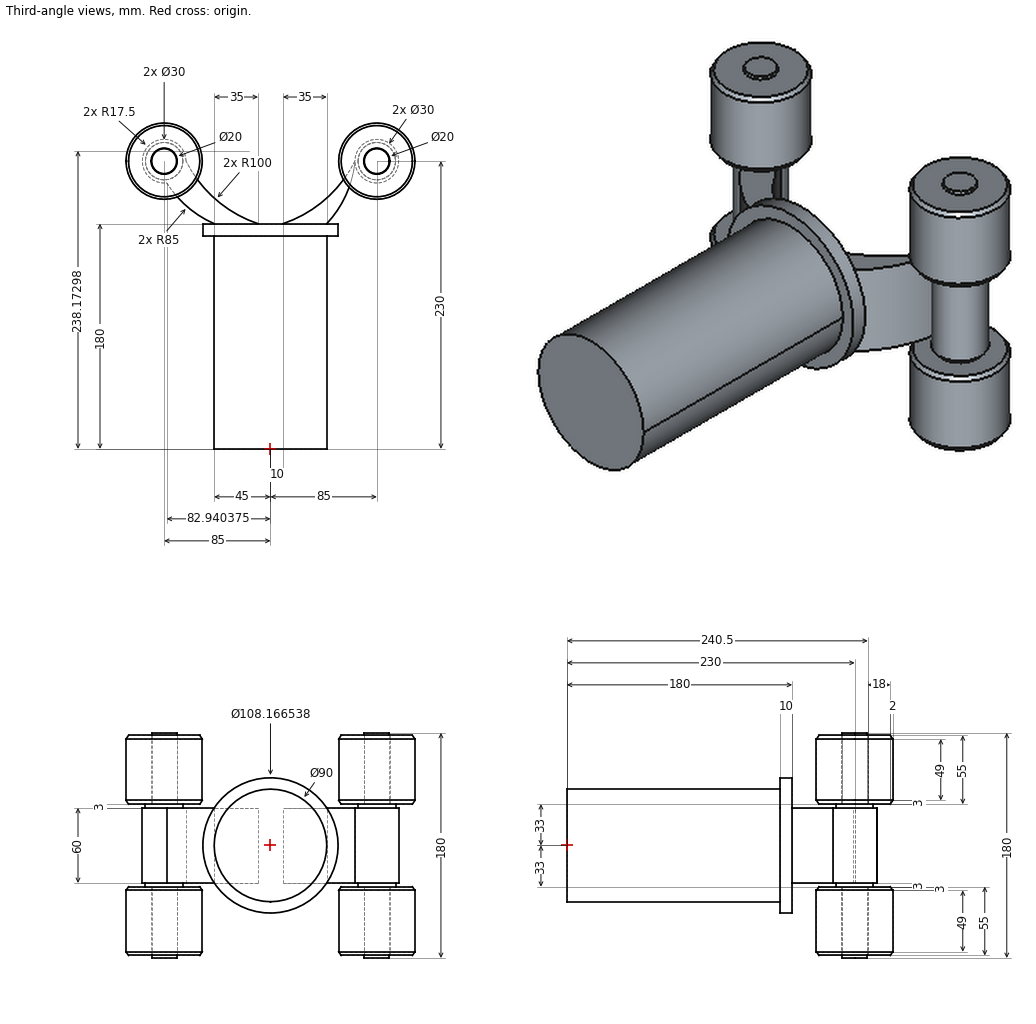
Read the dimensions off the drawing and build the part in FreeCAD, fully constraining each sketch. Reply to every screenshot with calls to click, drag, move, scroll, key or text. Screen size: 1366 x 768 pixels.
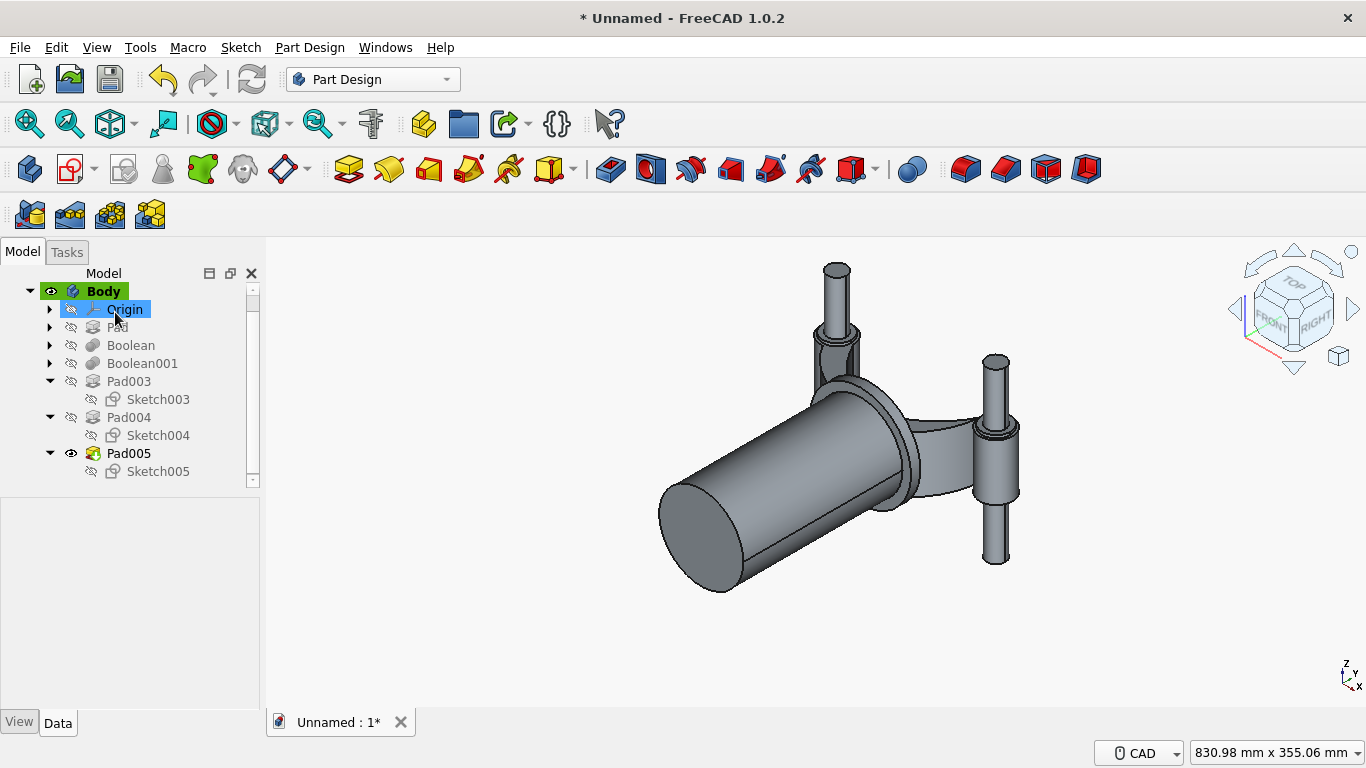
click(50, 309)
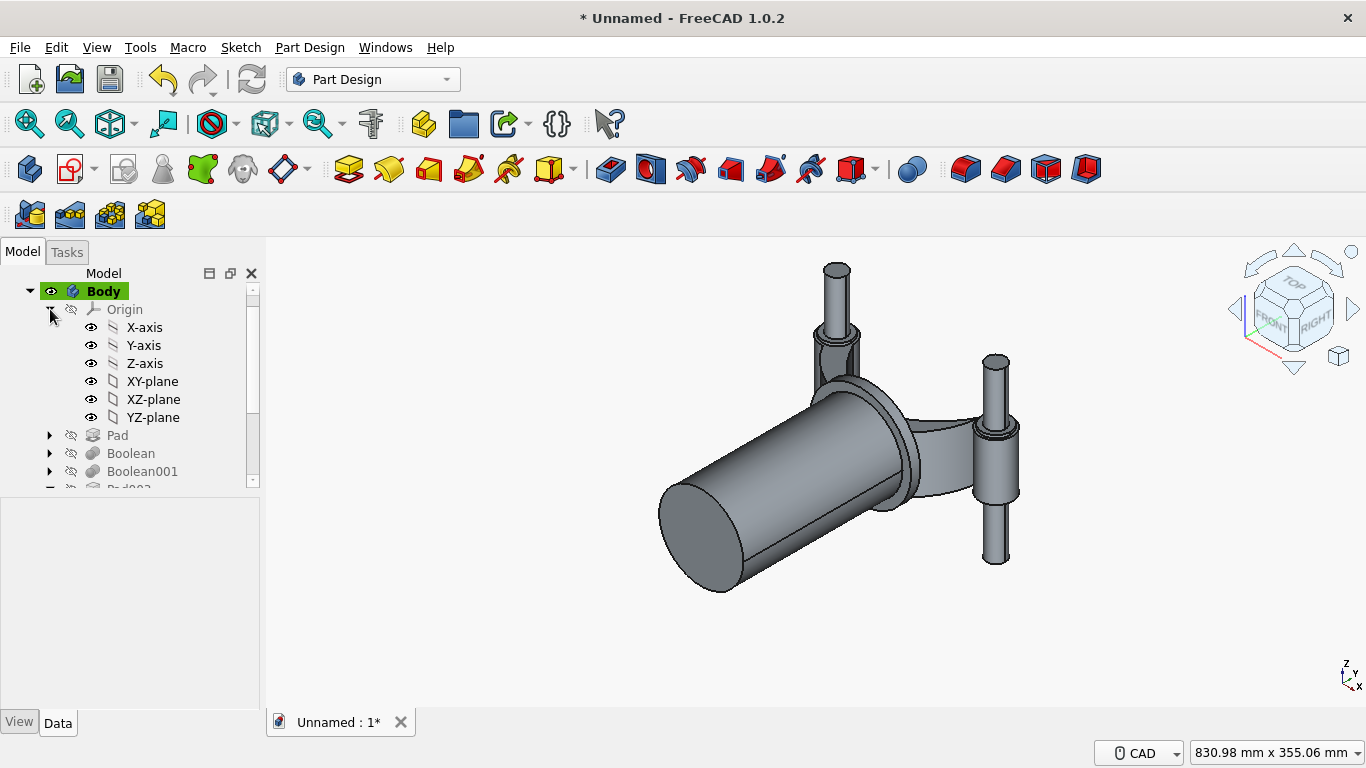
click(136, 381)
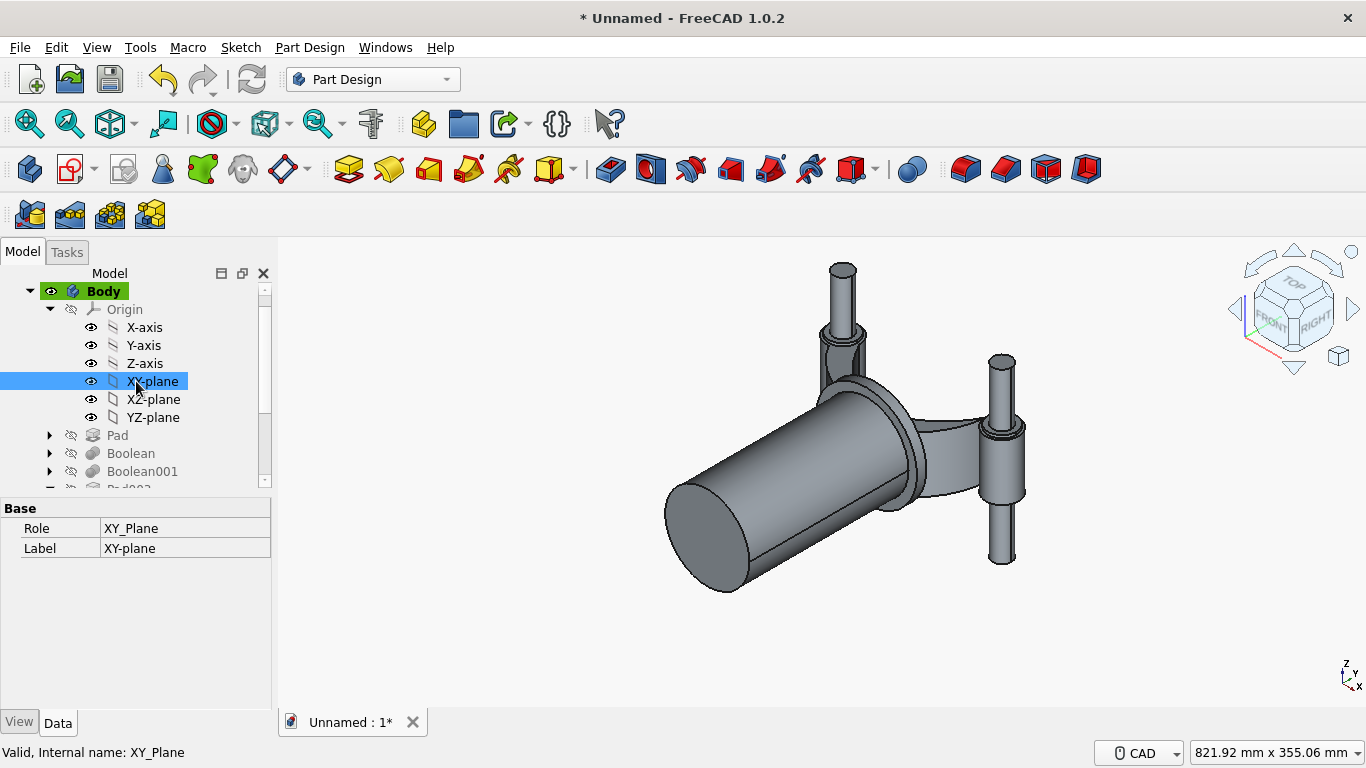
click(284, 170)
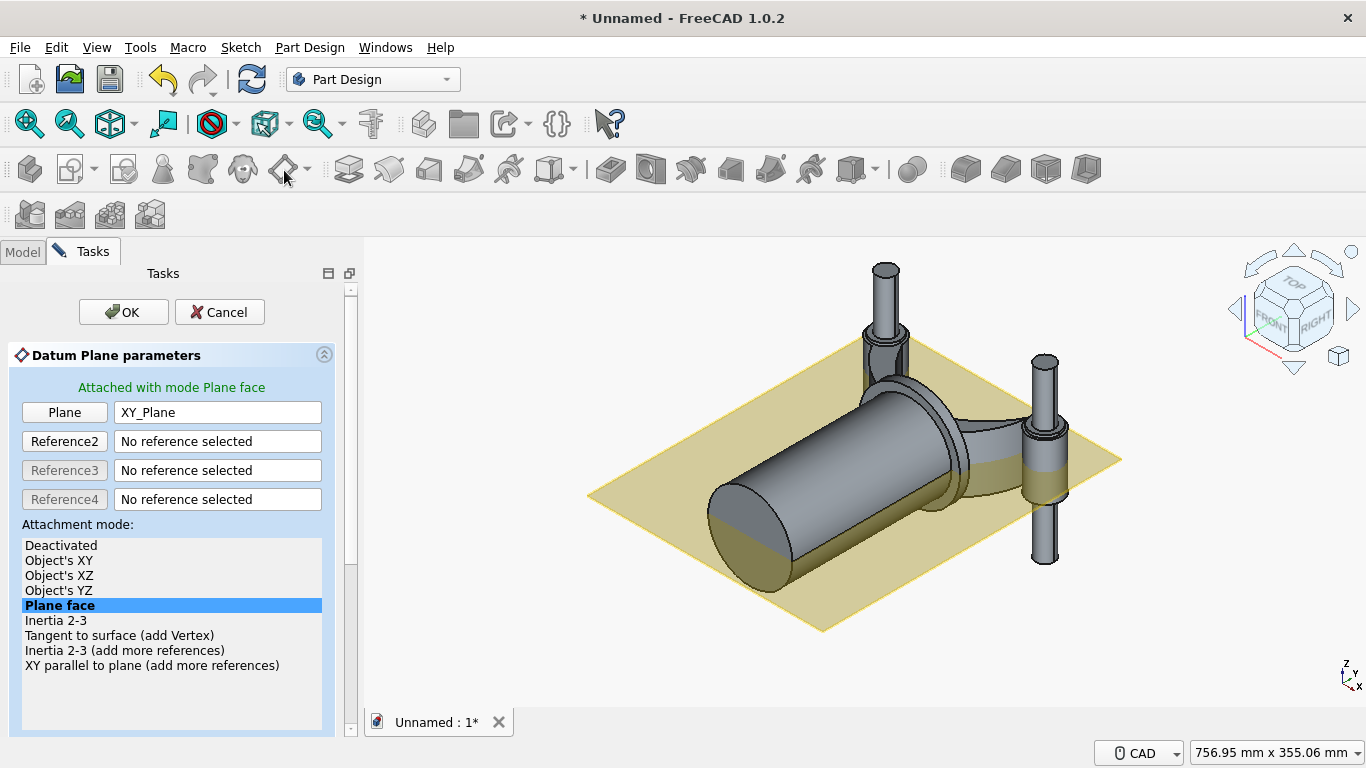
scroll(351, 510, down, 3)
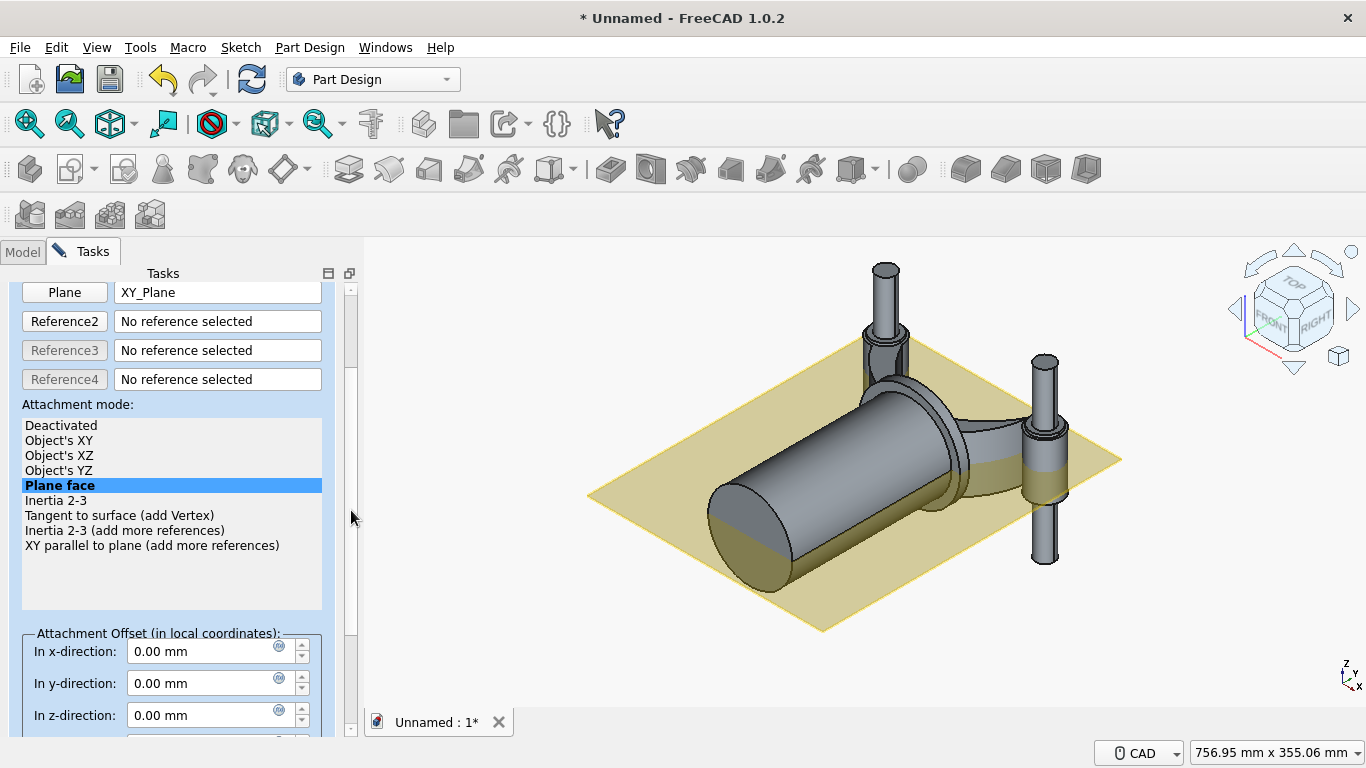
triple_click(210, 655)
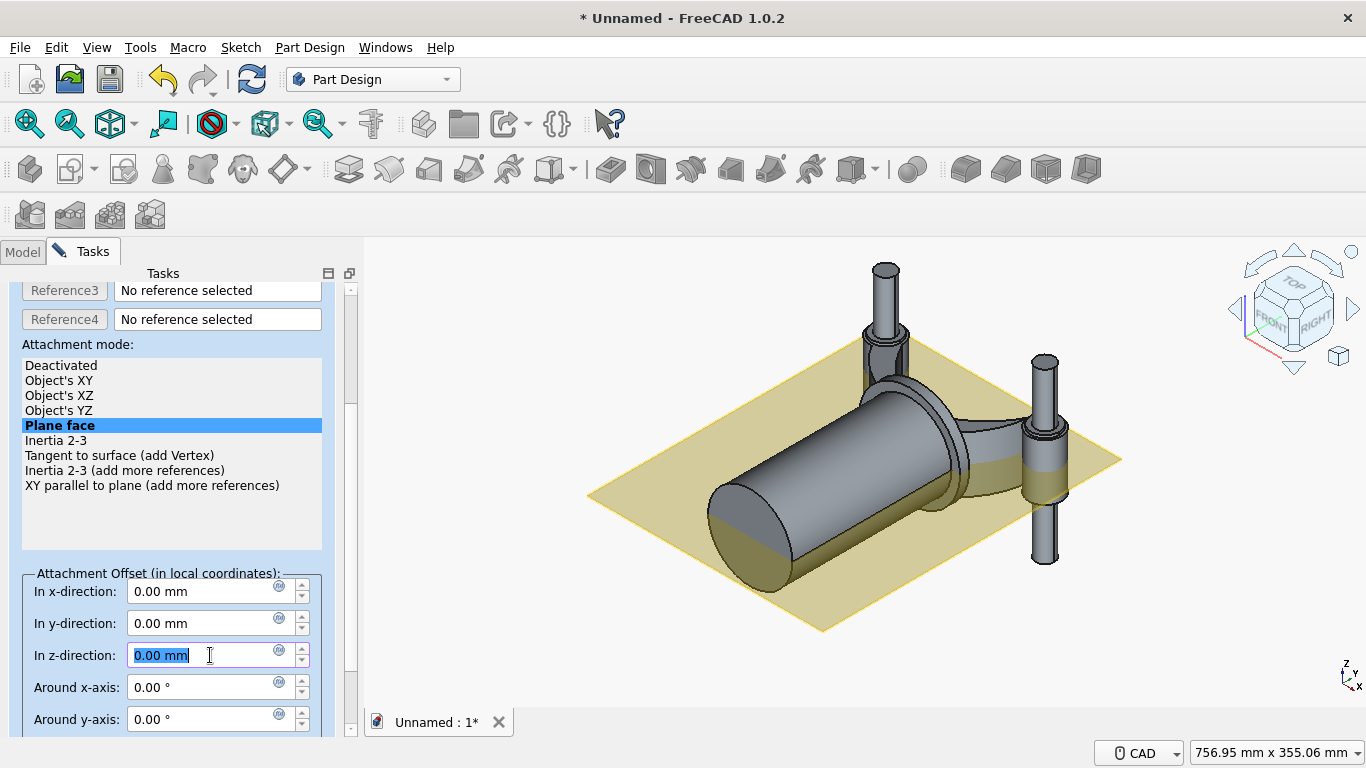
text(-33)
key(Tab)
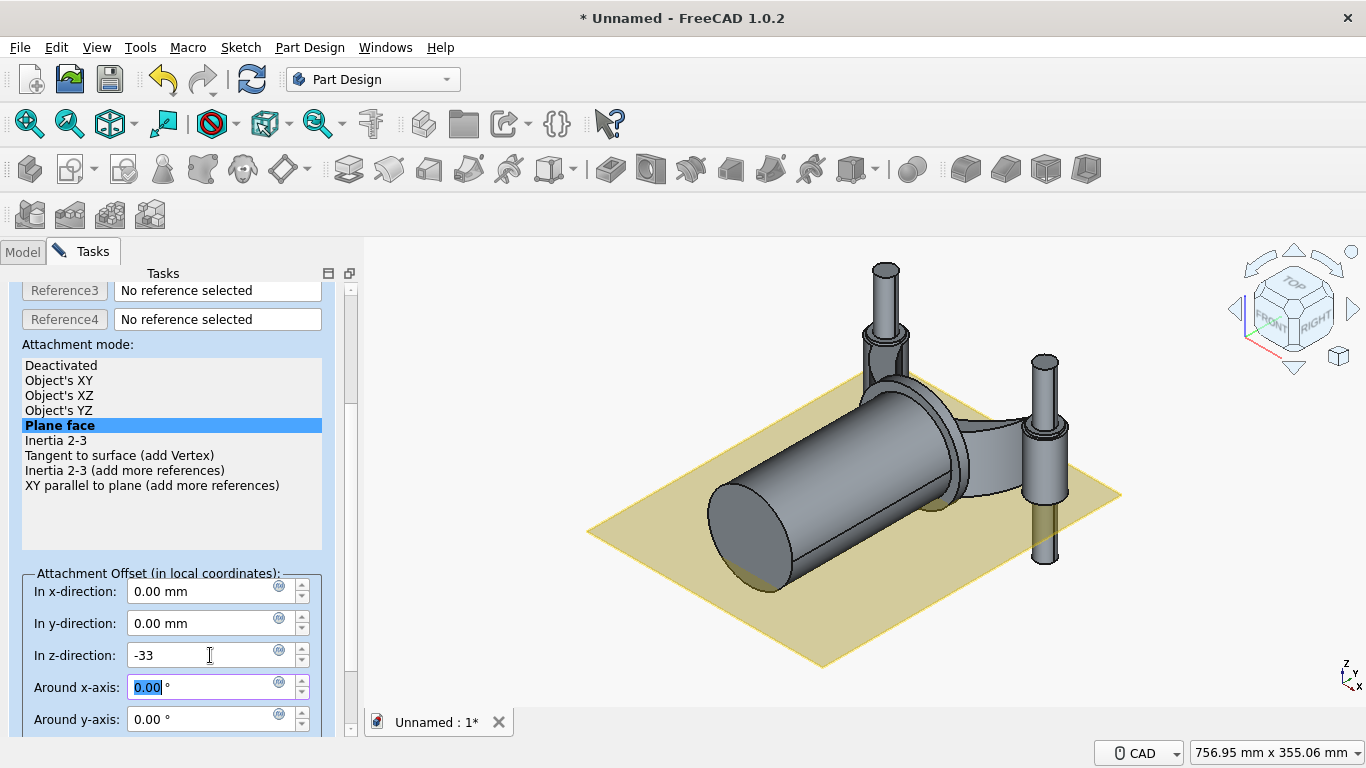
scroll(351, 510, up, 4)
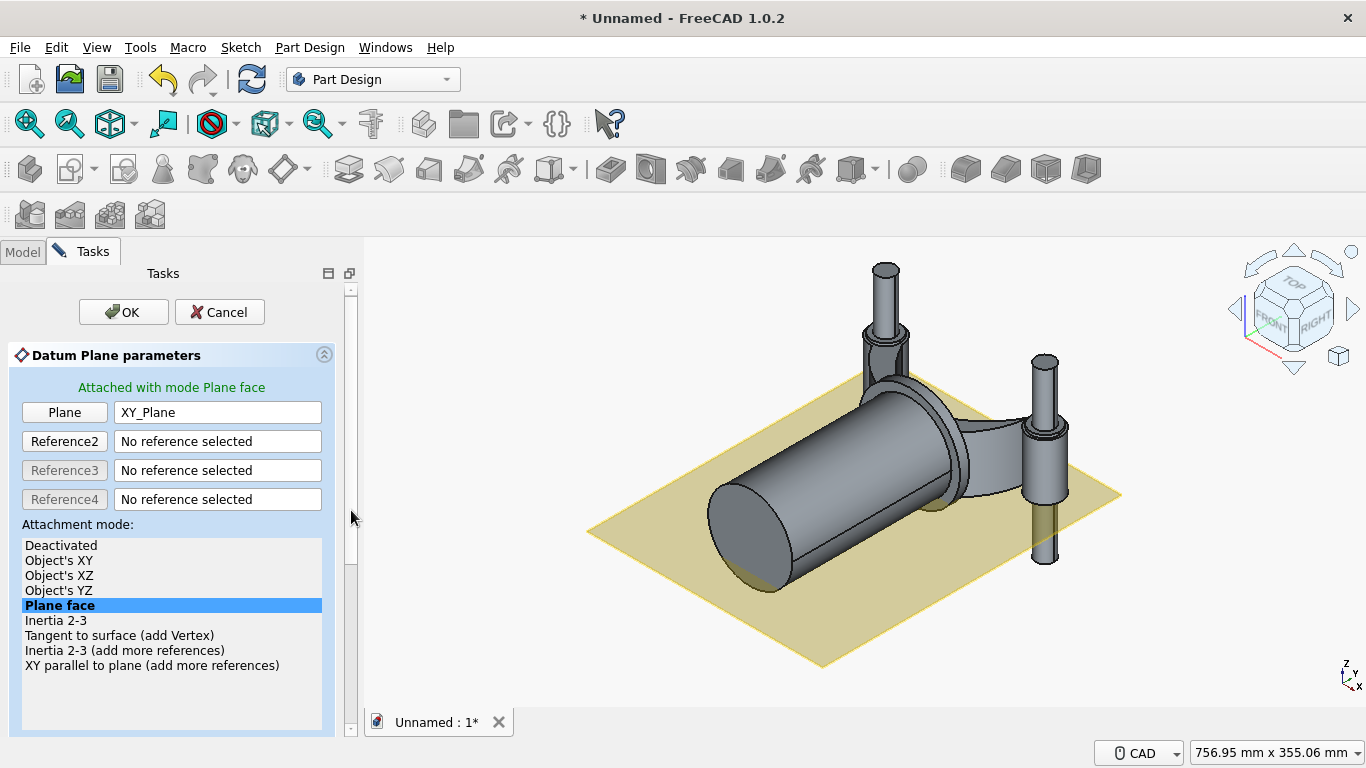
click(124, 312)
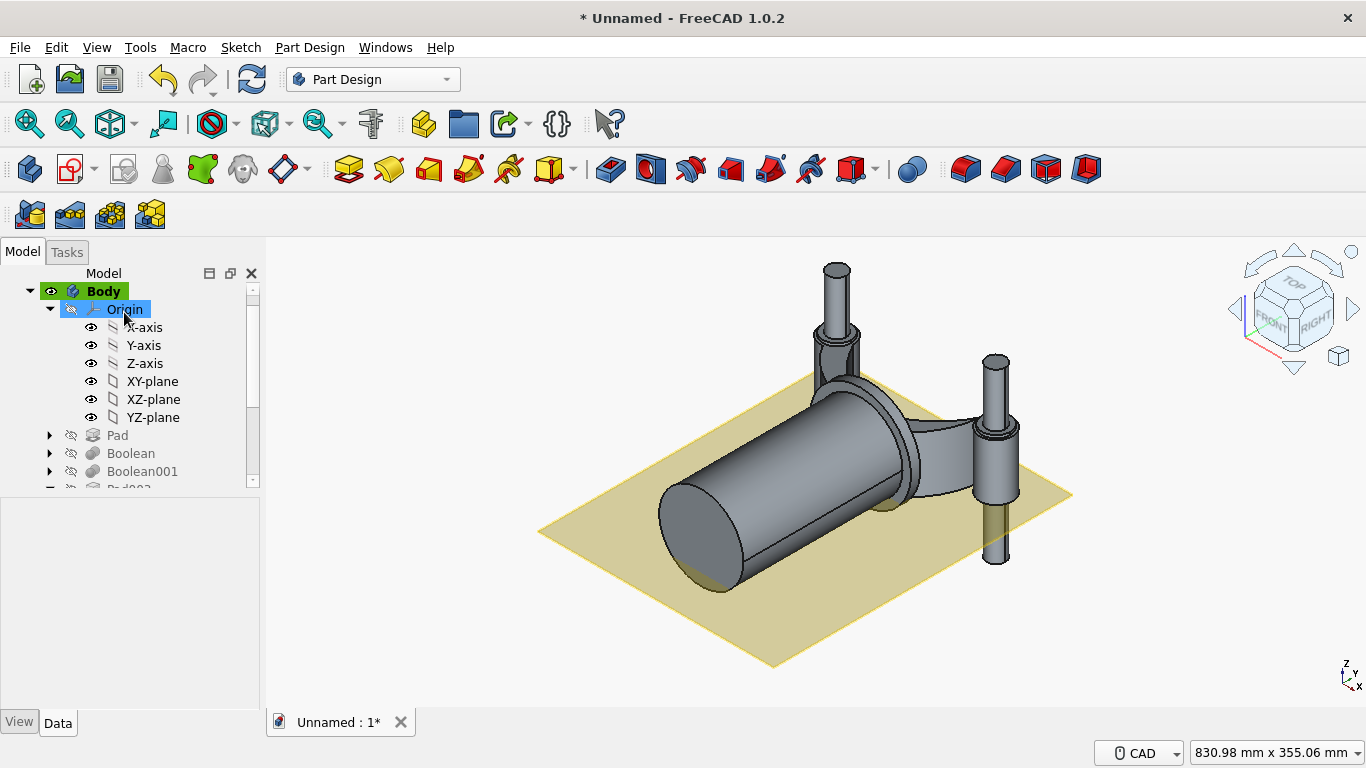
scroll(120, 377, down, 3)